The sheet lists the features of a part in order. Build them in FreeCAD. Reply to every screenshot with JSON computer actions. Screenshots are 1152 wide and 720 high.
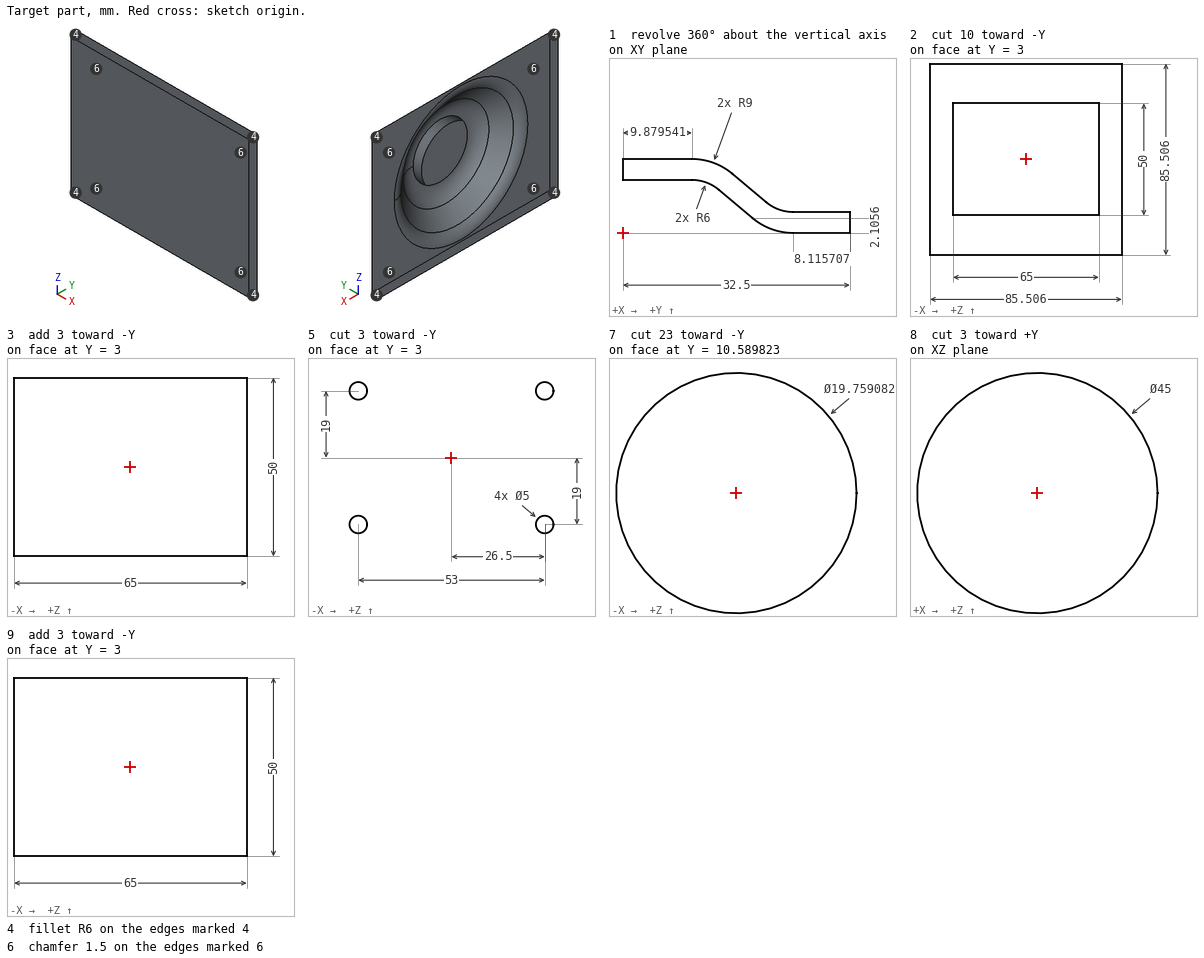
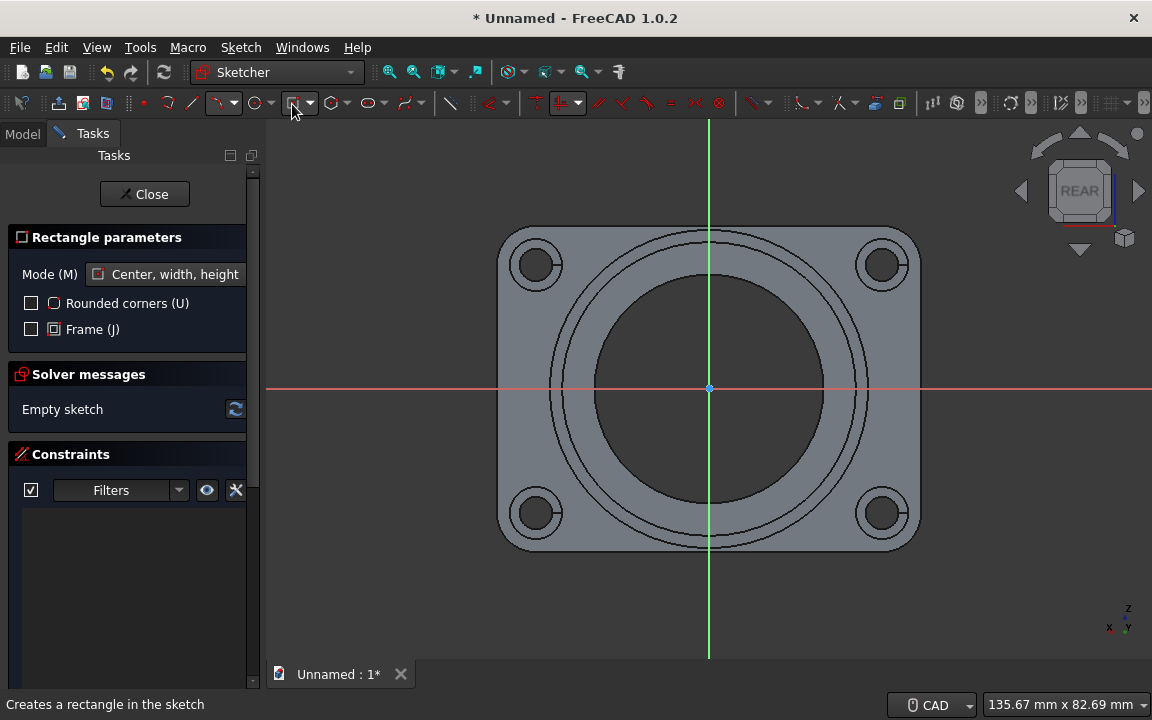
{"action": "left_click", "coordinate": [709, 389]}
{"action": "left_click", "coordinate": [921, 226]}
{"action": "key", "text": "Escape"}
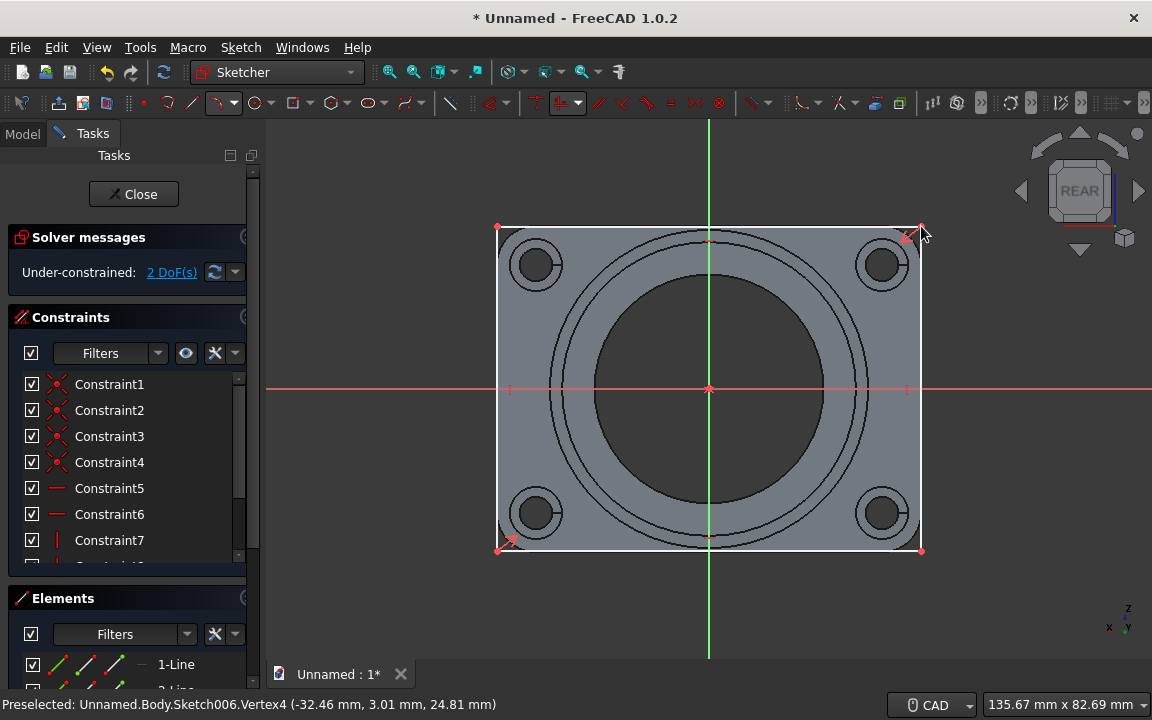
{"action": "left_click", "coordinate": [490, 104]}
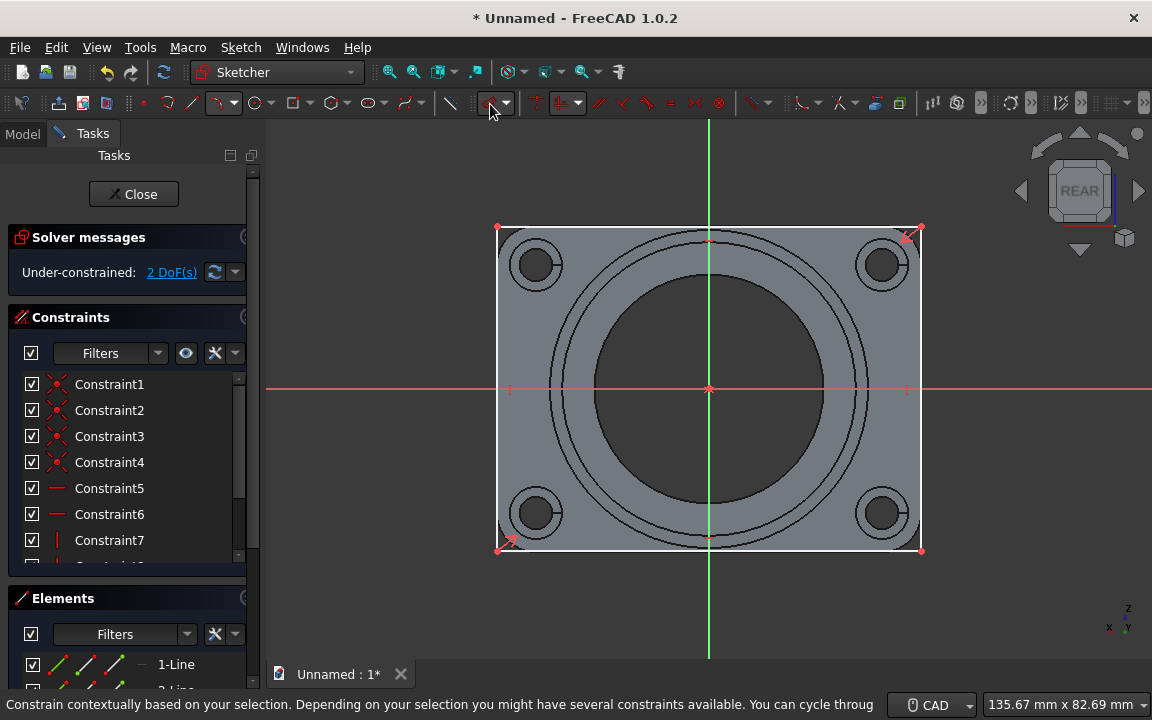
{"action": "left_click", "coordinate": [624, 551]}
{"action": "left_click", "coordinate": [611, 585]}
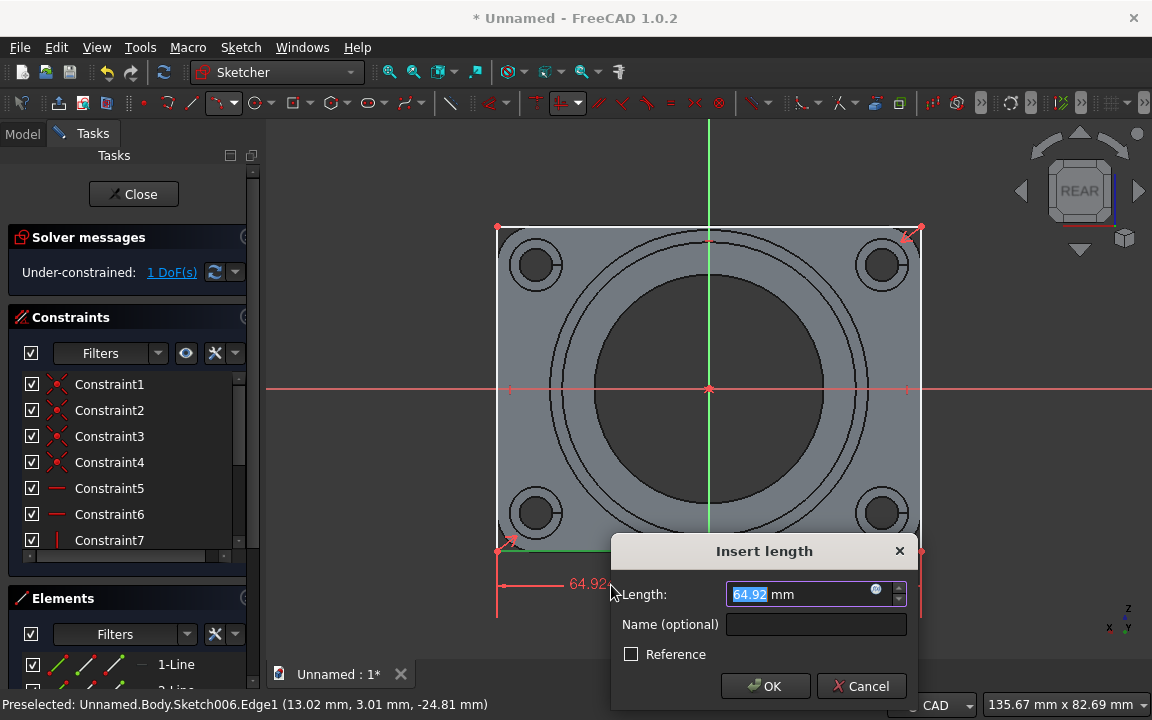
{"action": "type", "text": "65"}
{"action": "key", "text": "Return"}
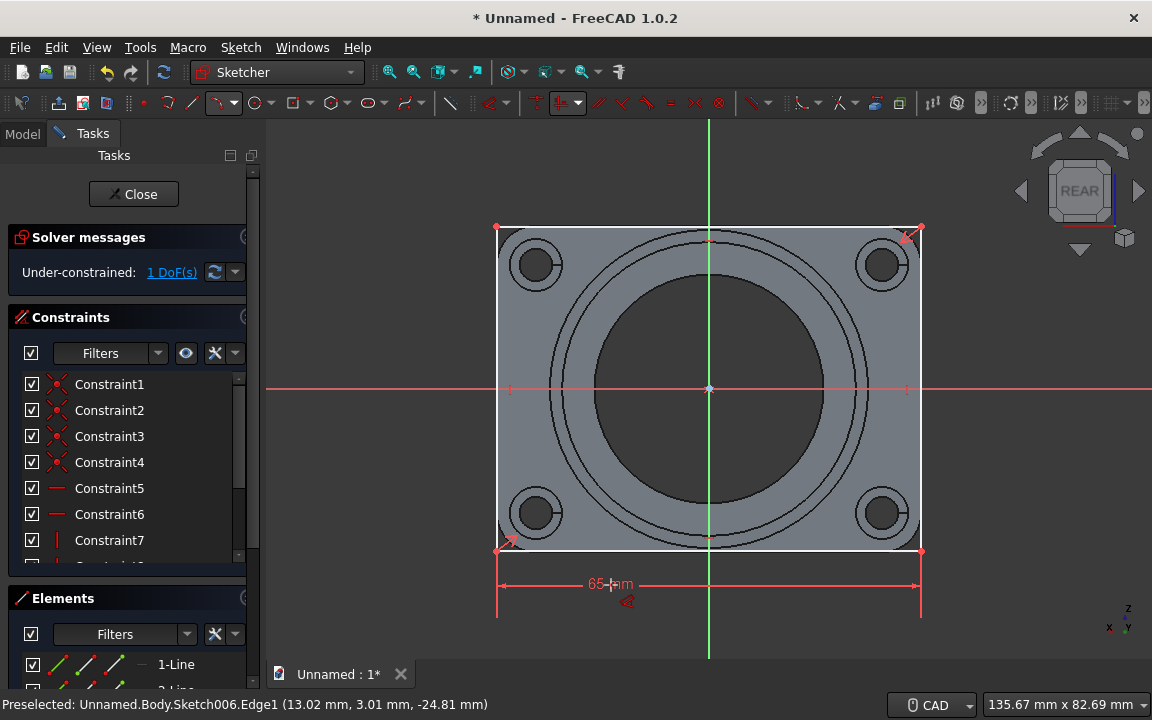
{"action": "left_click", "coordinate": [921, 454]}
{"action": "left_click", "coordinate": [955, 314]}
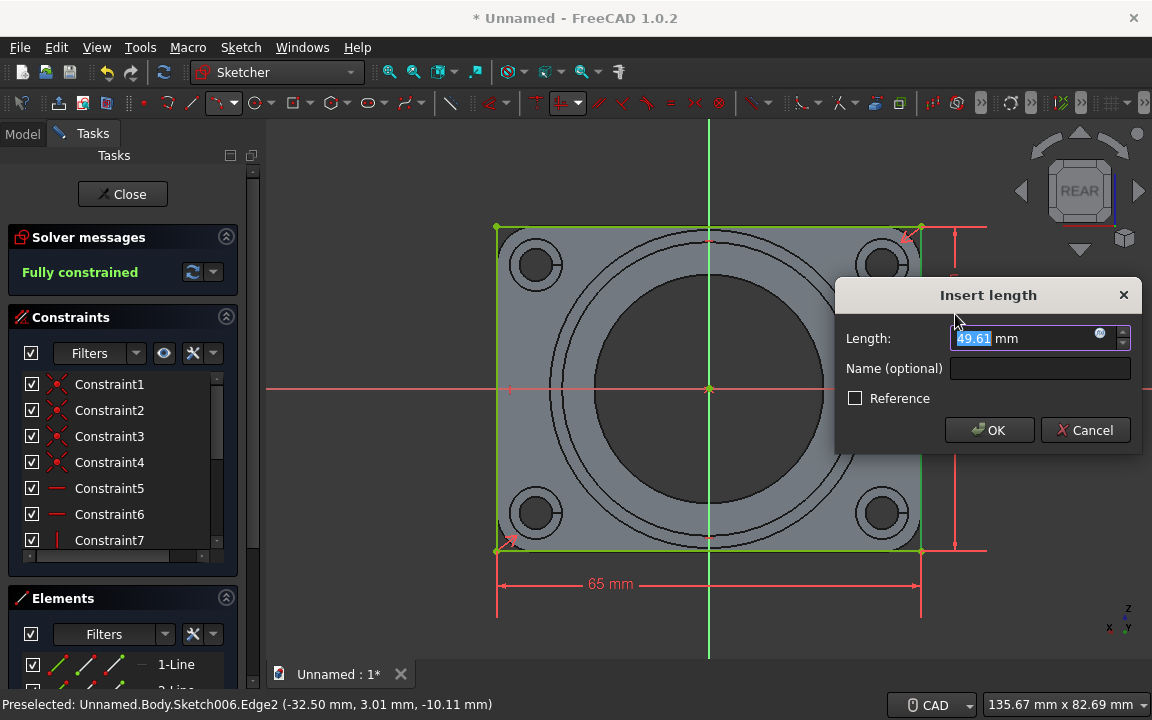
{"action": "type", "text": "50"}
{"action": "key", "text": "Return"}
{"action": "key", "text": "Escape"}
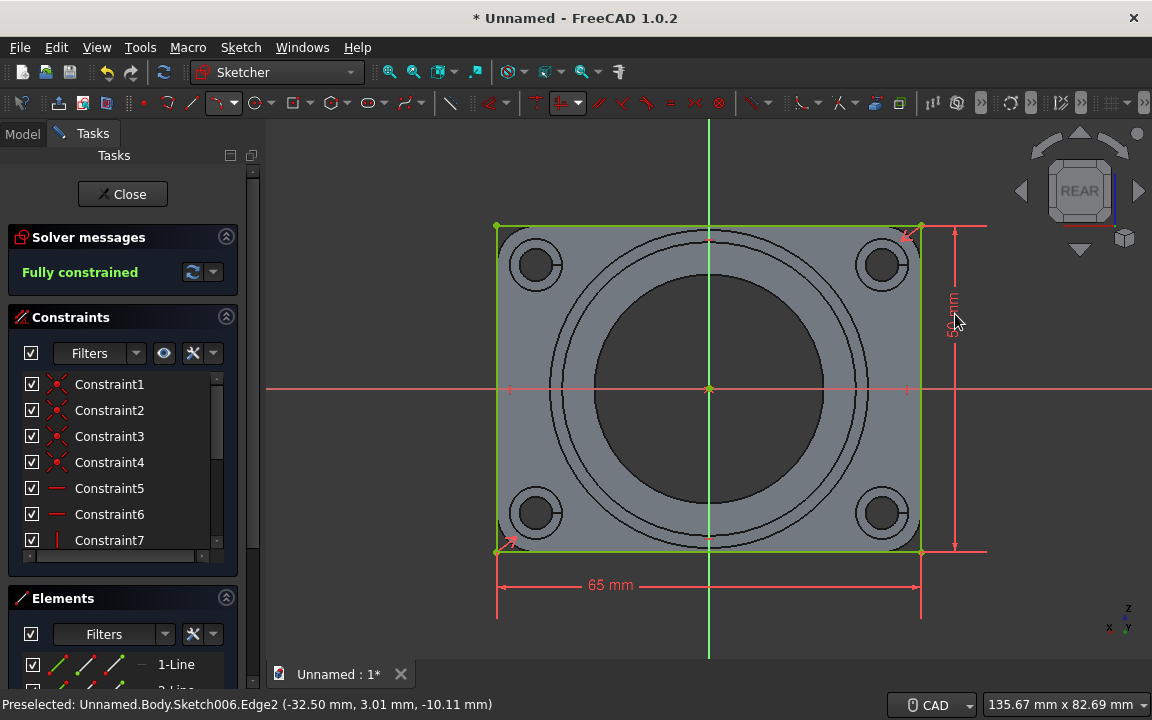
{"action": "left_click", "coordinate": [123, 194]}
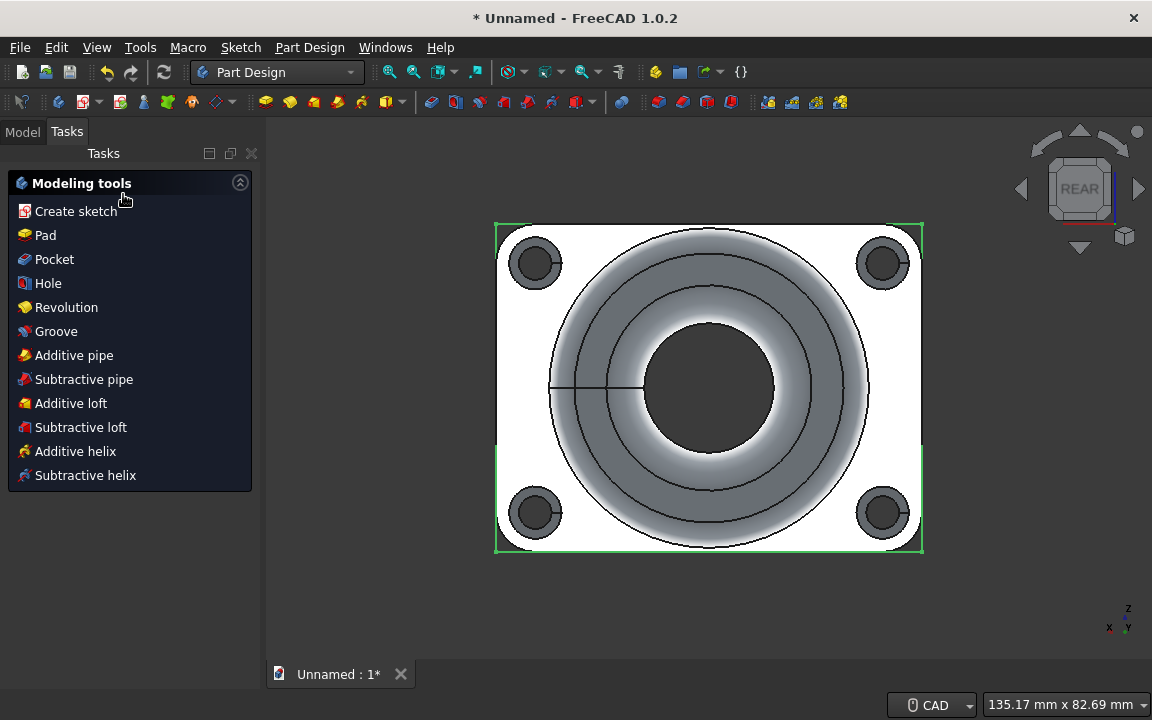
{"action": "left_click", "coordinate": [266, 102]}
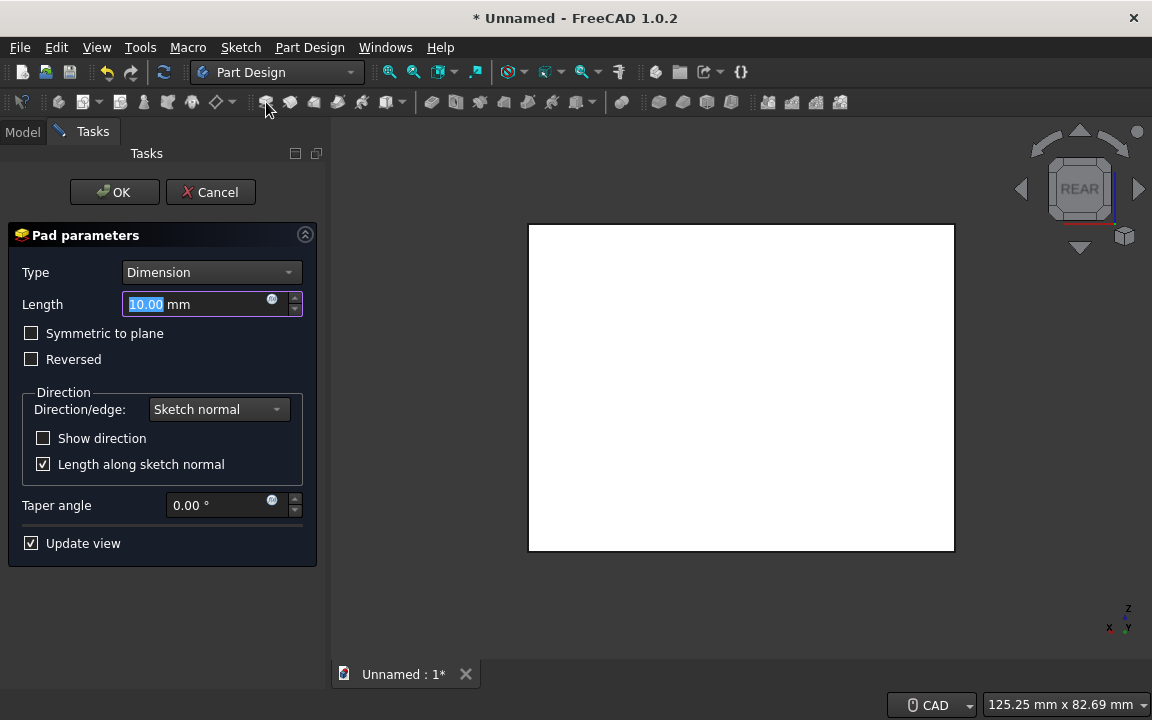
{"action": "type", "text": "3"}
{"action": "key", "text": "Tab"}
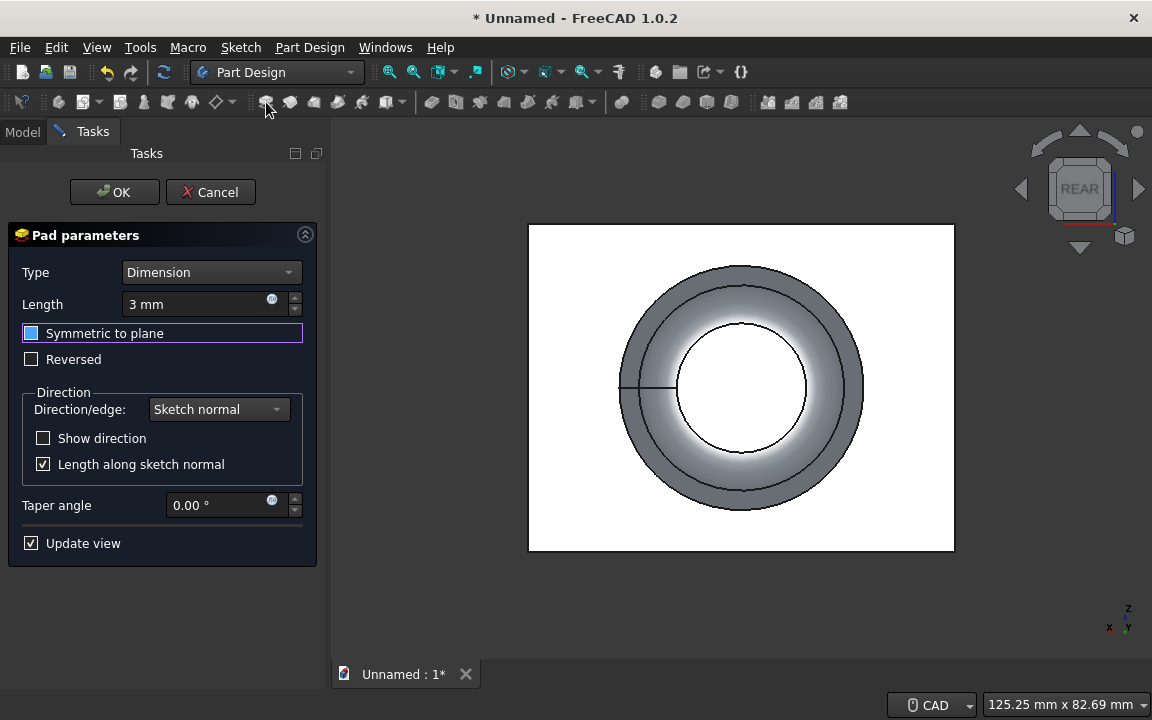
{"action": "left_click", "coordinate": [30, 359]}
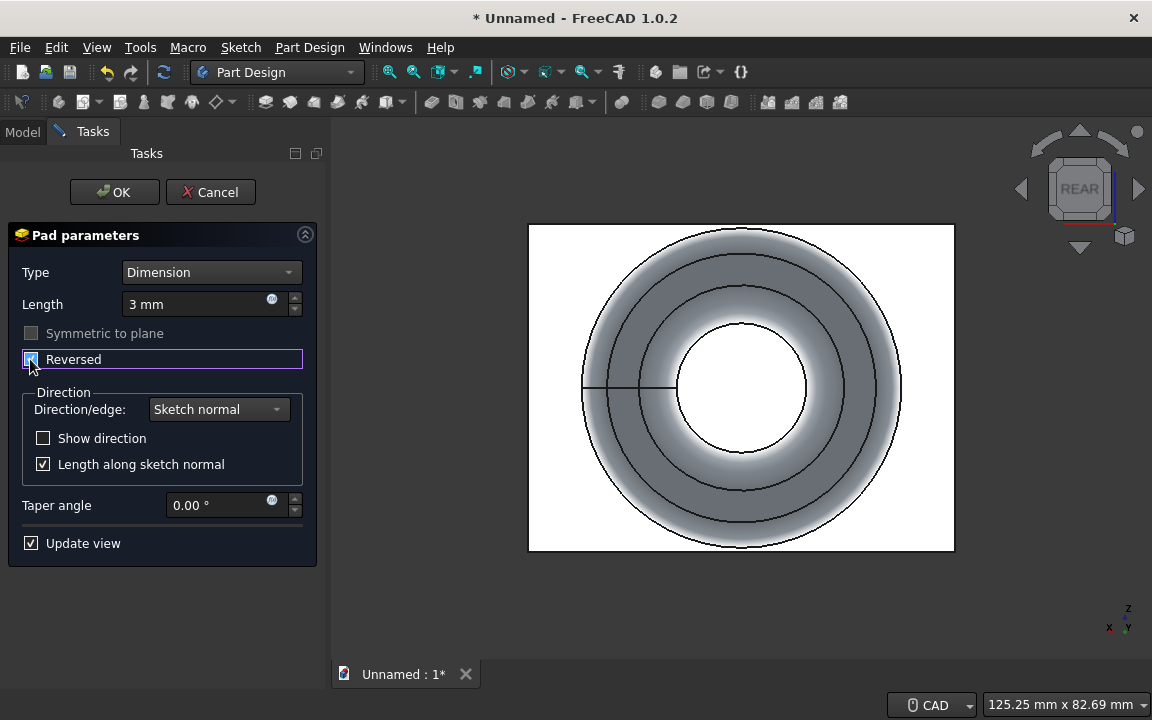
{"action": "left_click", "coordinate": [115, 192]}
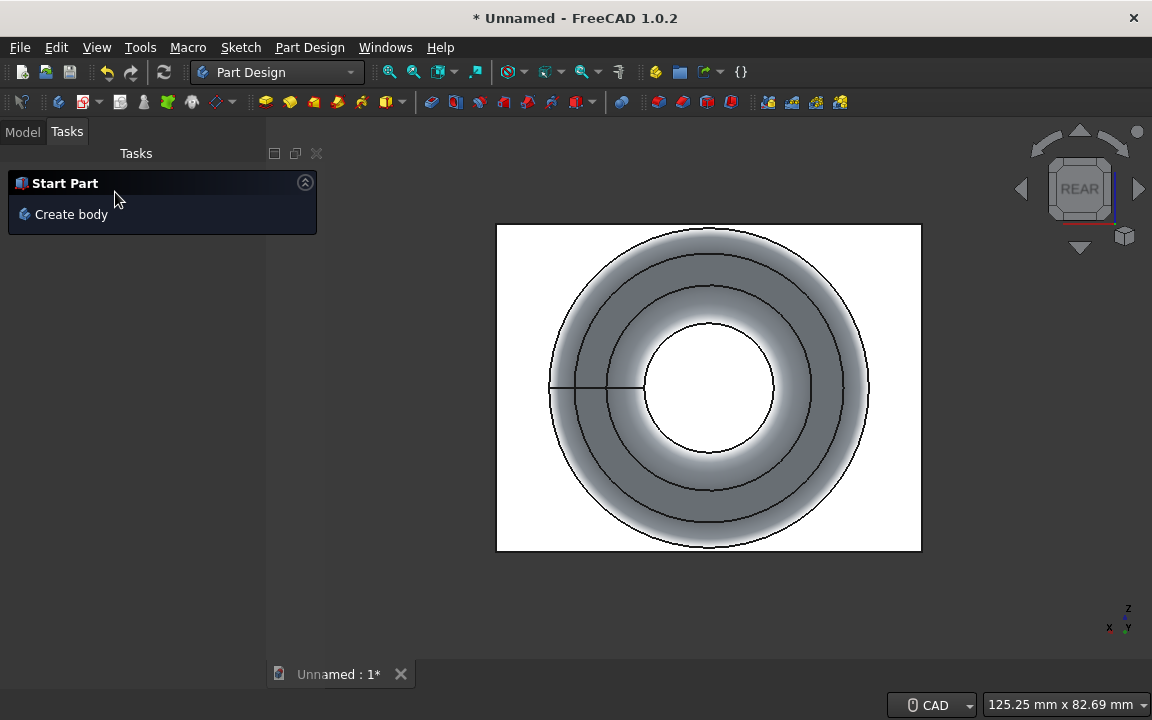
{"action": "key", "text": "0"}